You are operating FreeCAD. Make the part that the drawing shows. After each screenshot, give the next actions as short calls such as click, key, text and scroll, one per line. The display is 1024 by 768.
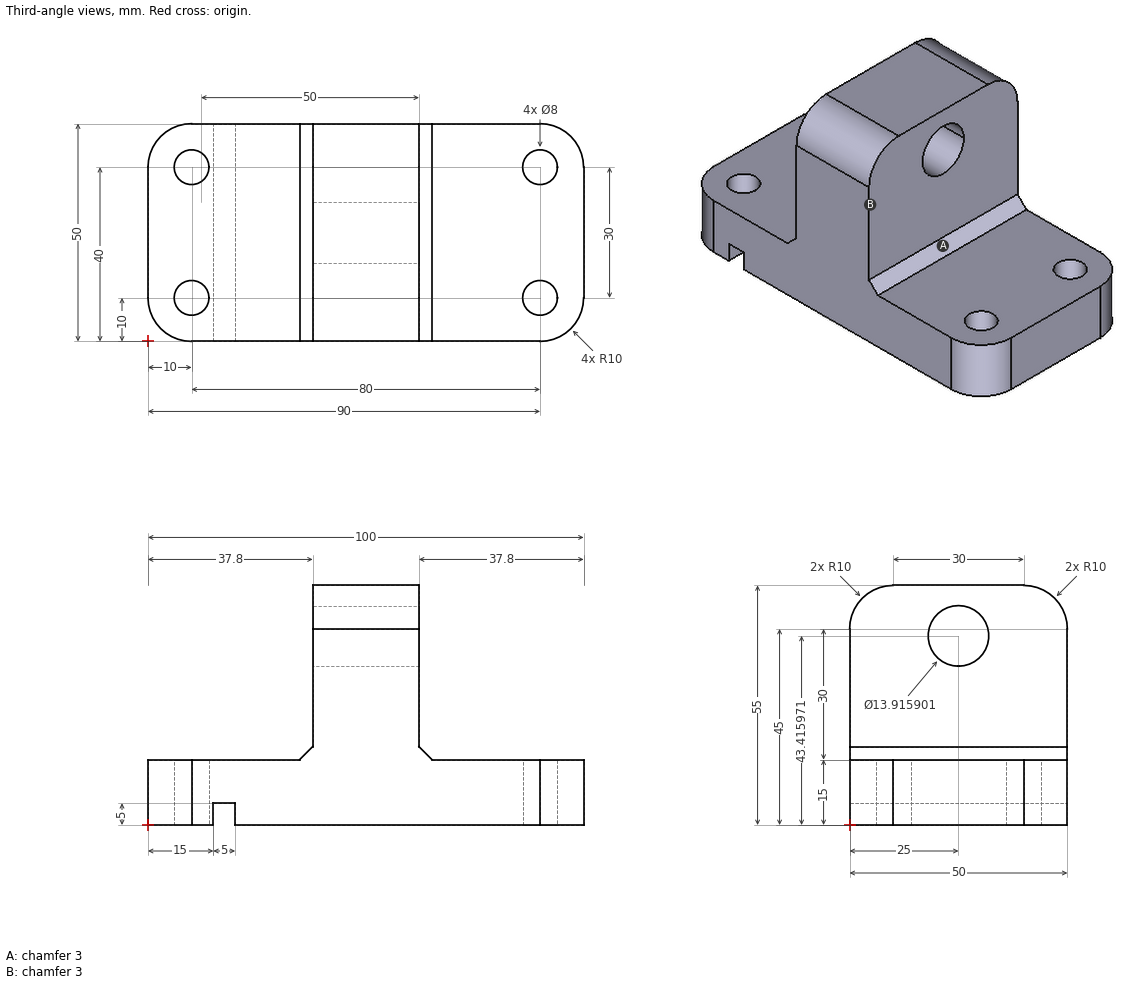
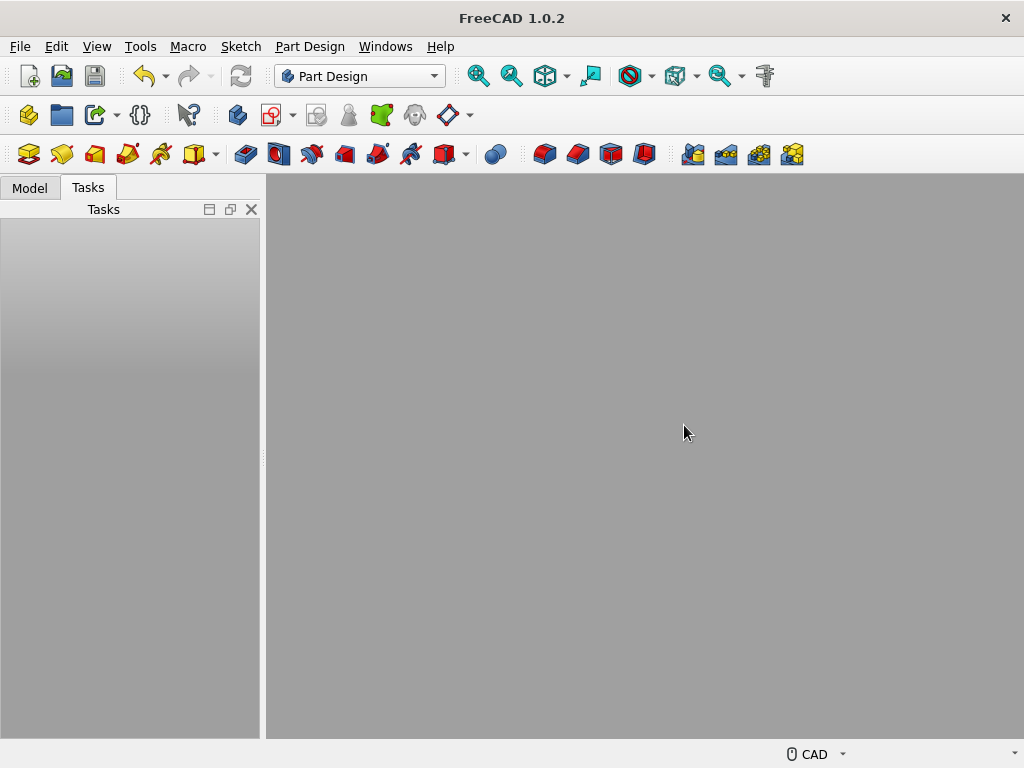
click(29, 76)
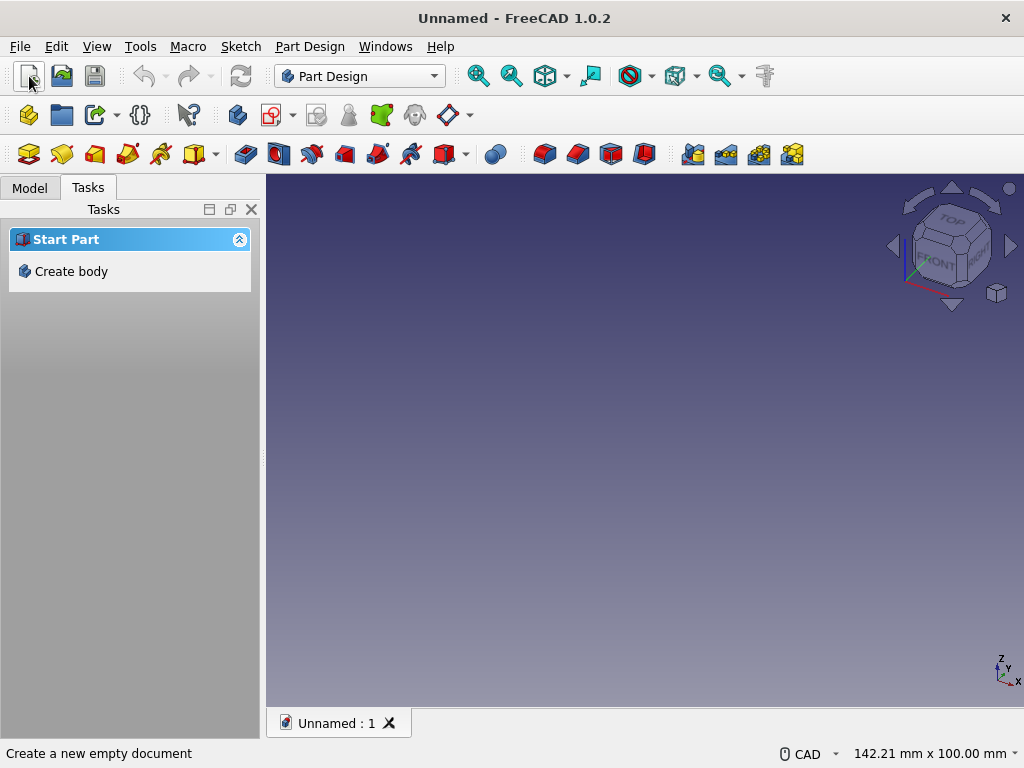
click(270, 116)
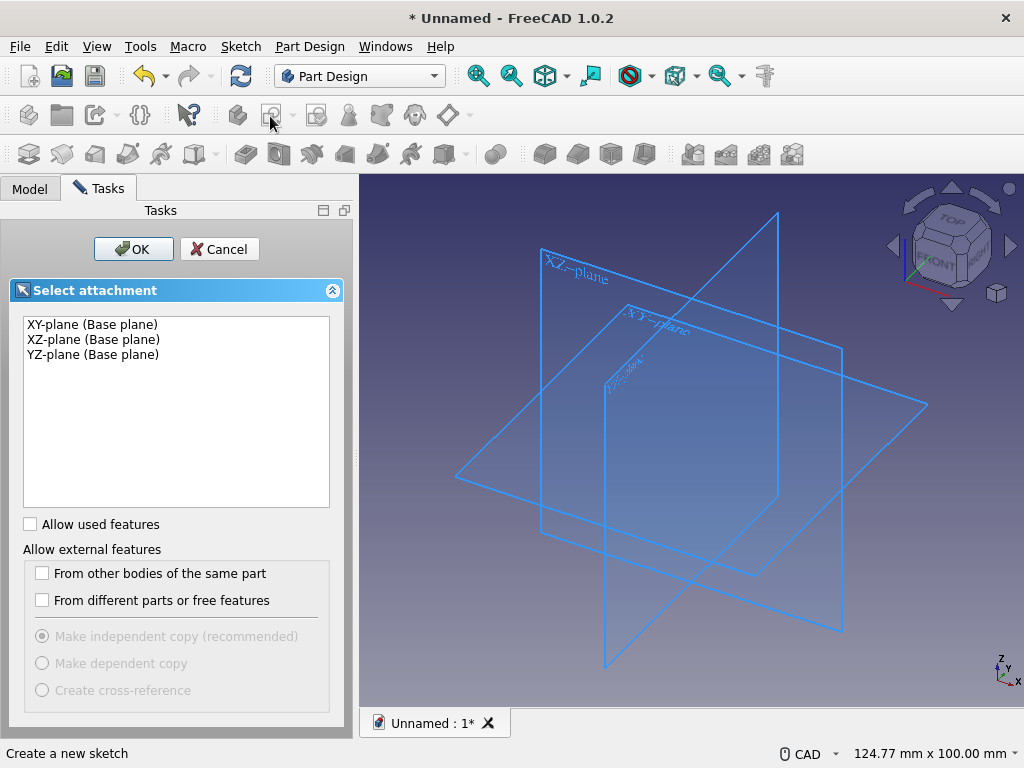
click(84, 324)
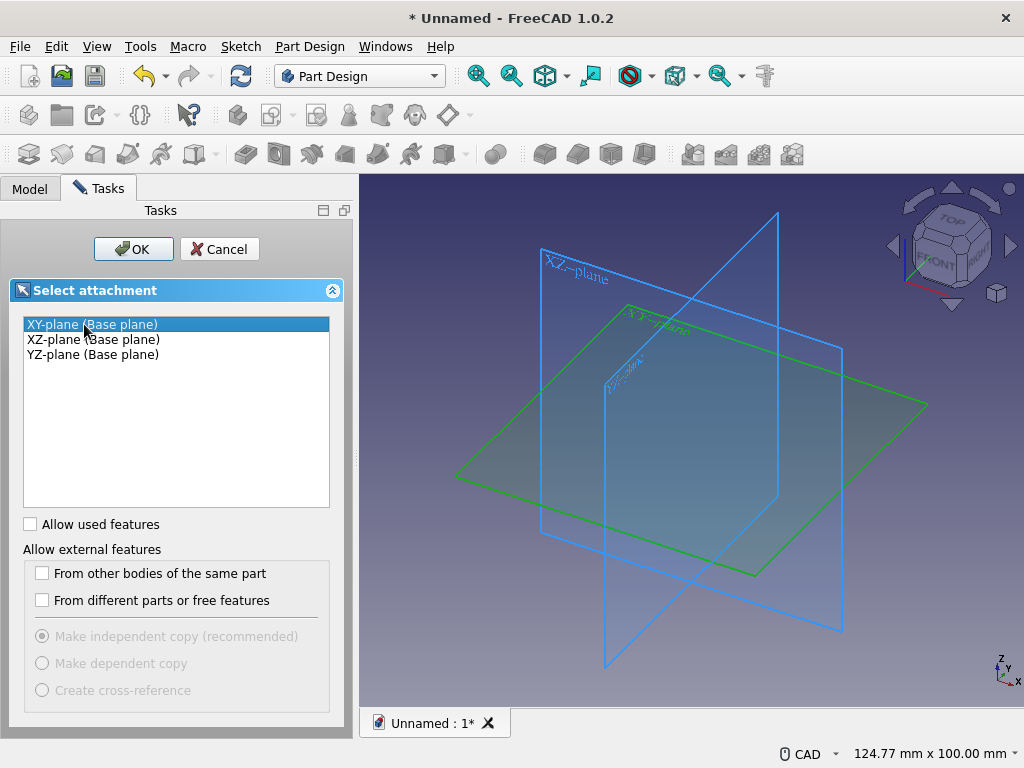
click(134, 249)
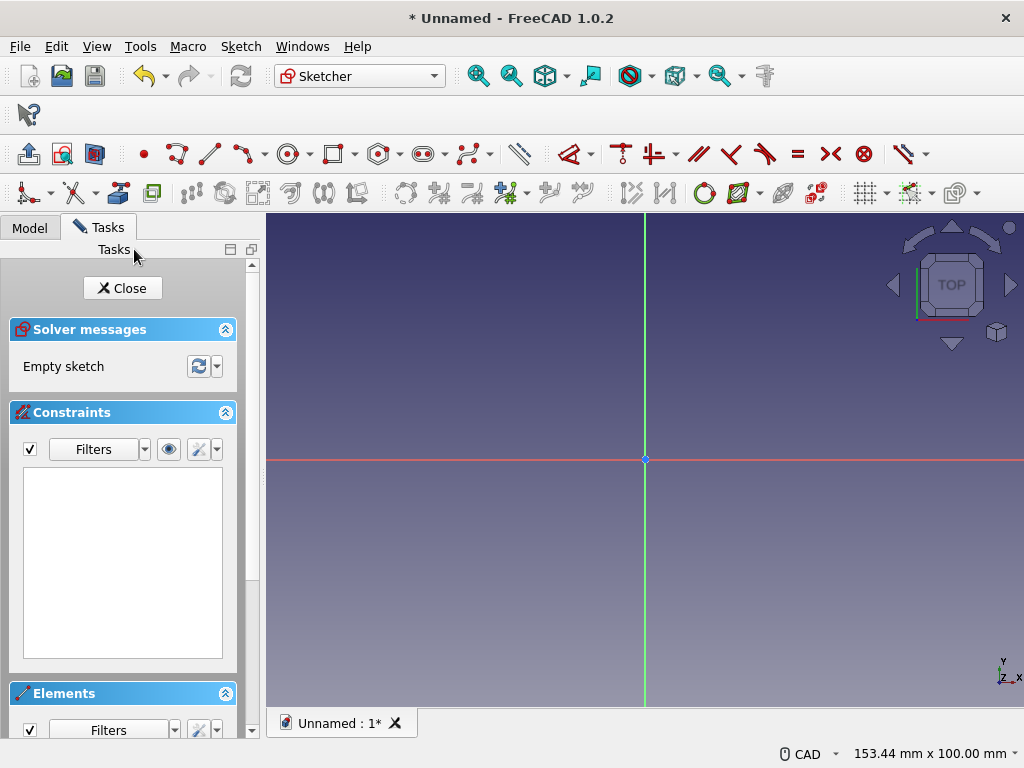
scroll(294, 610, down, 3)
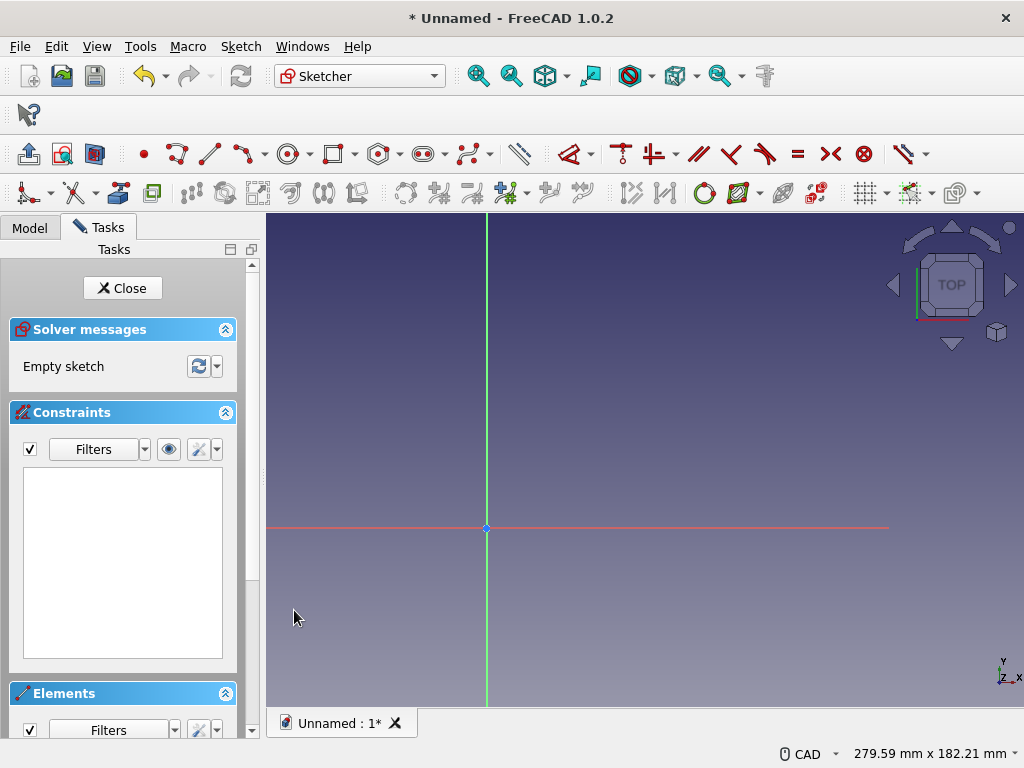
scroll(715, 461, up, 2)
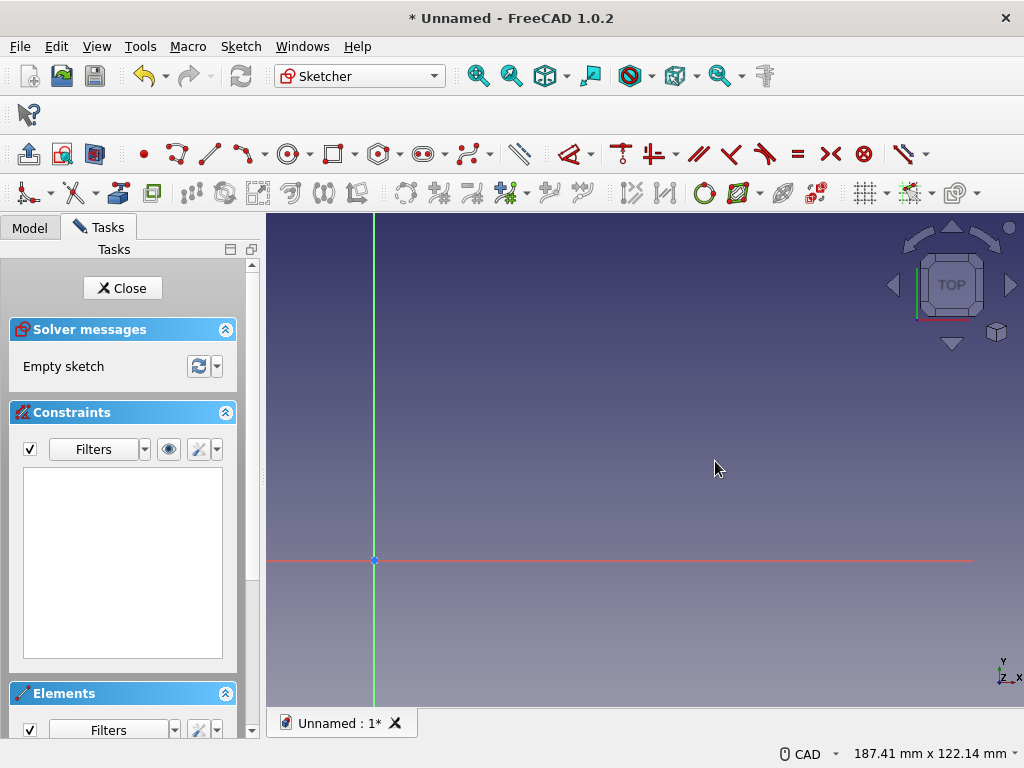
click(210, 154)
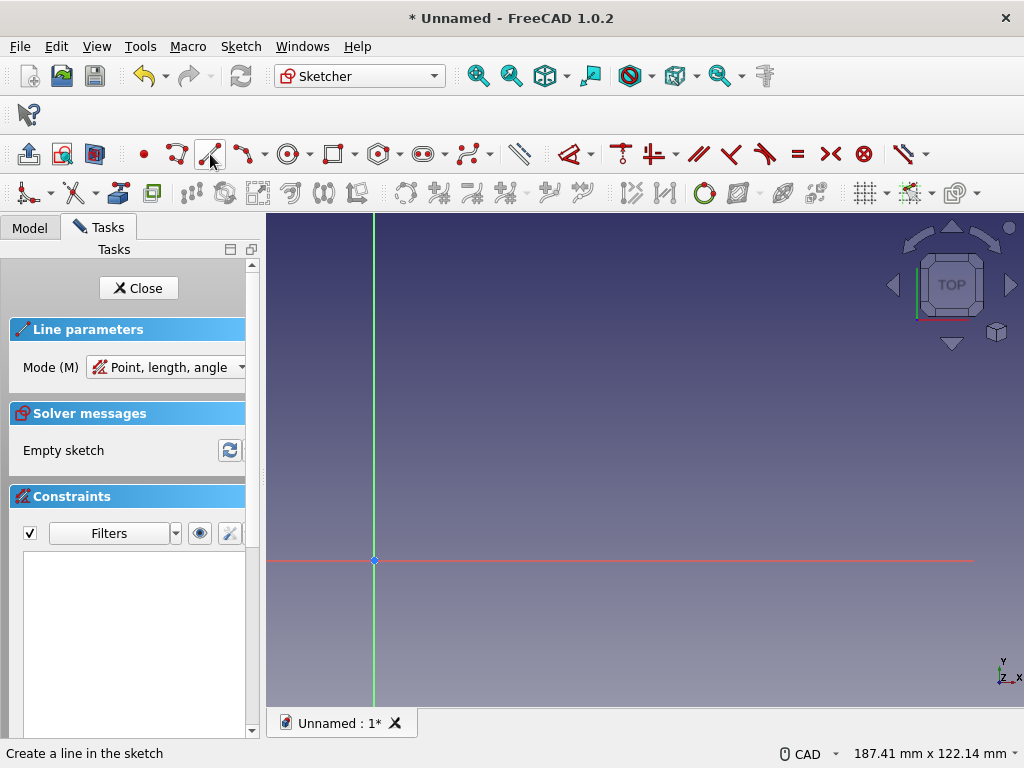
click(414, 561)
click(738, 552)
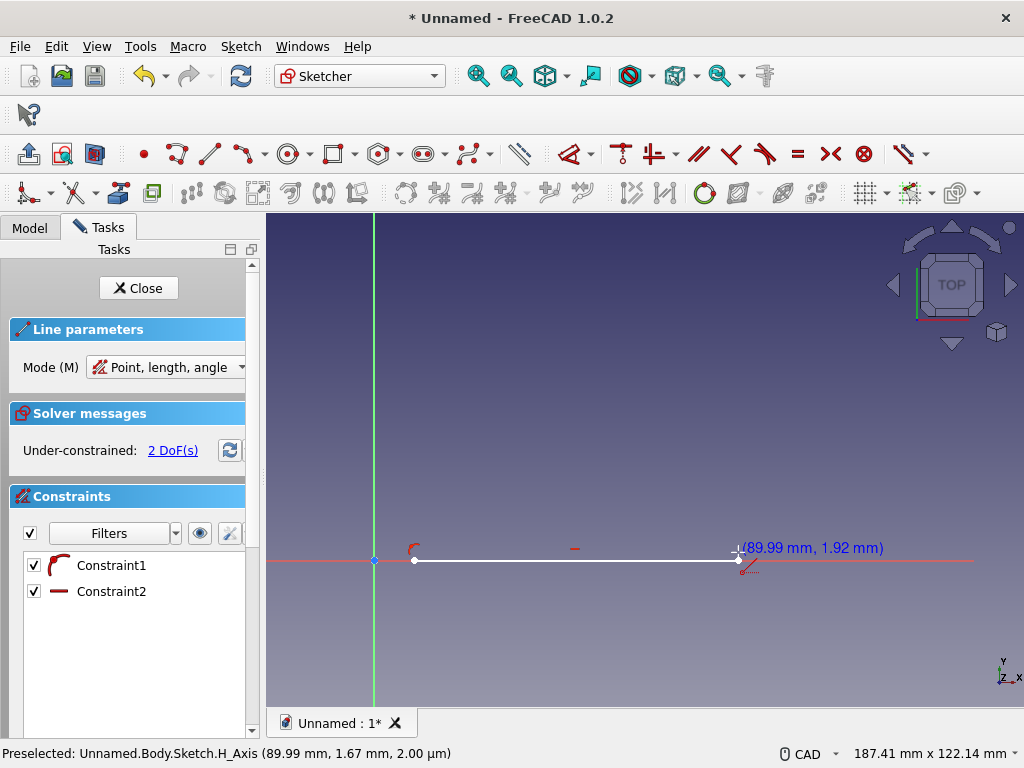
click(779, 520)
click(779, 399)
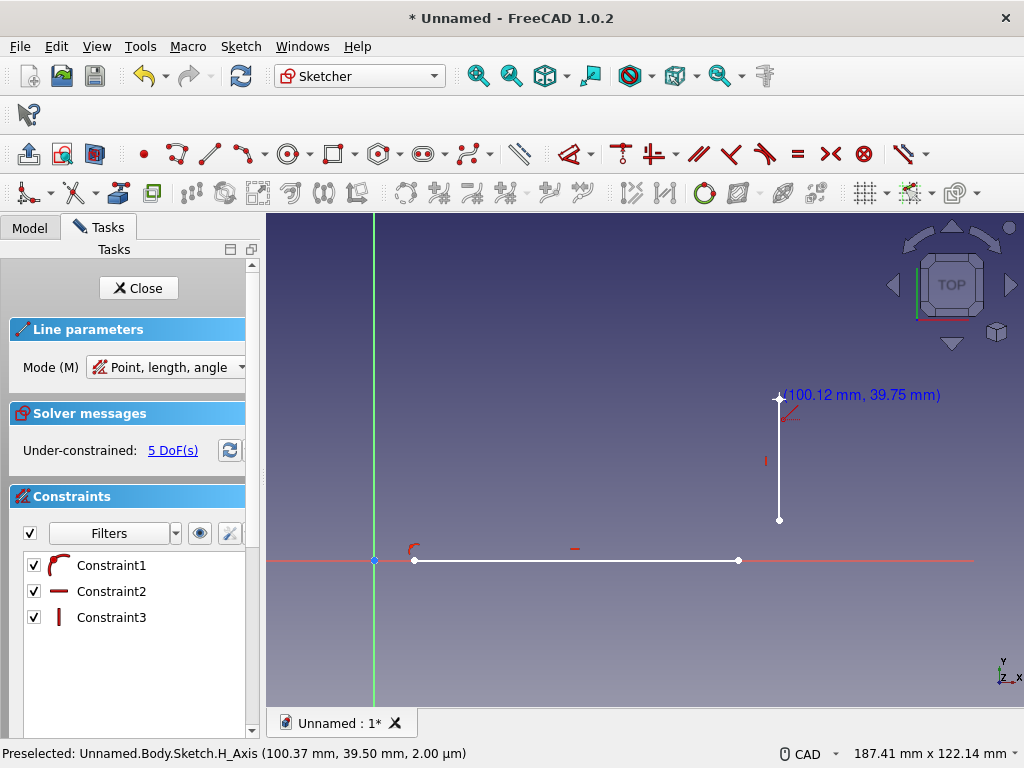
click(738, 359)
click(414, 359)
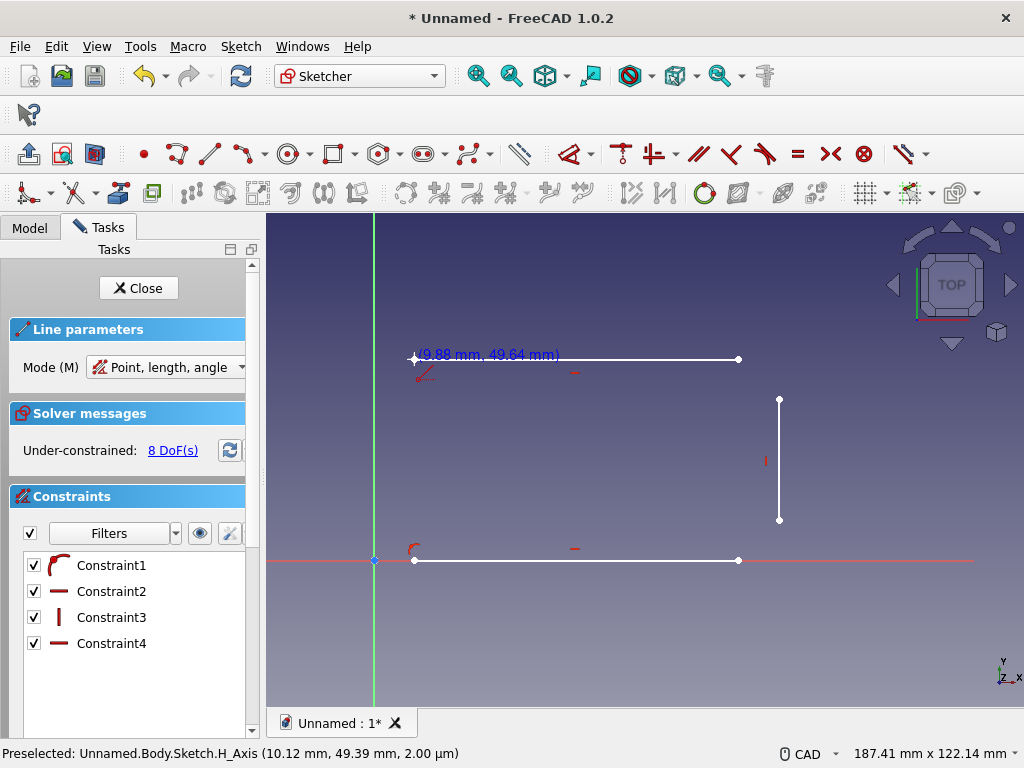
click(374, 399)
click(383, 520)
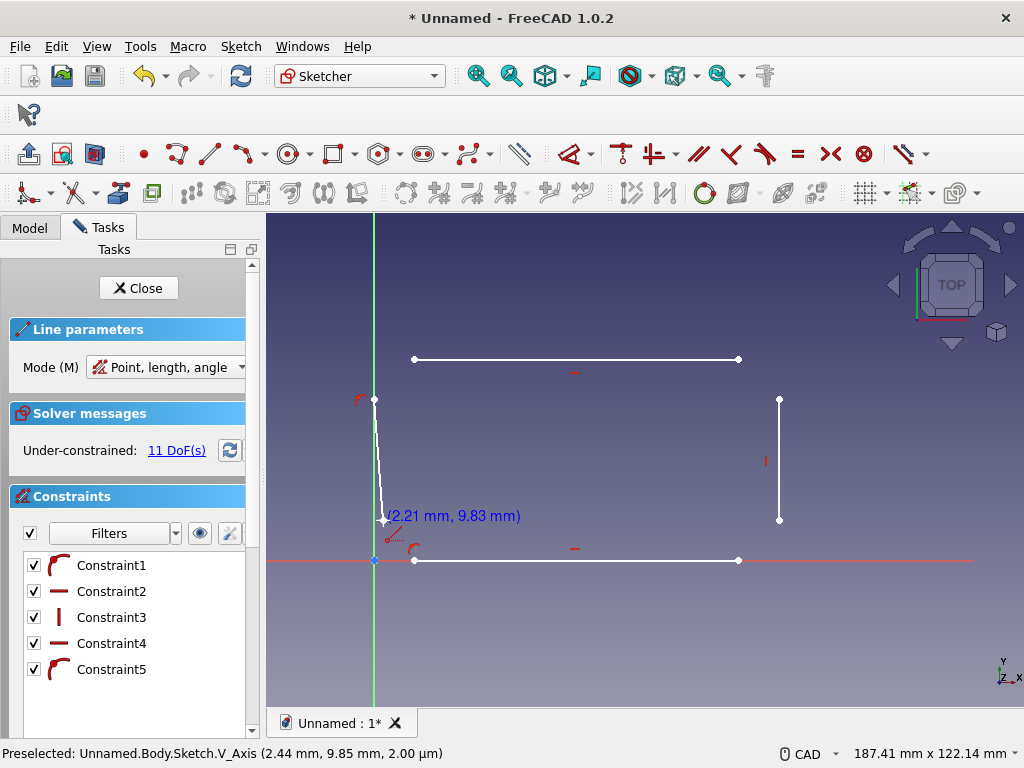
click(242, 154)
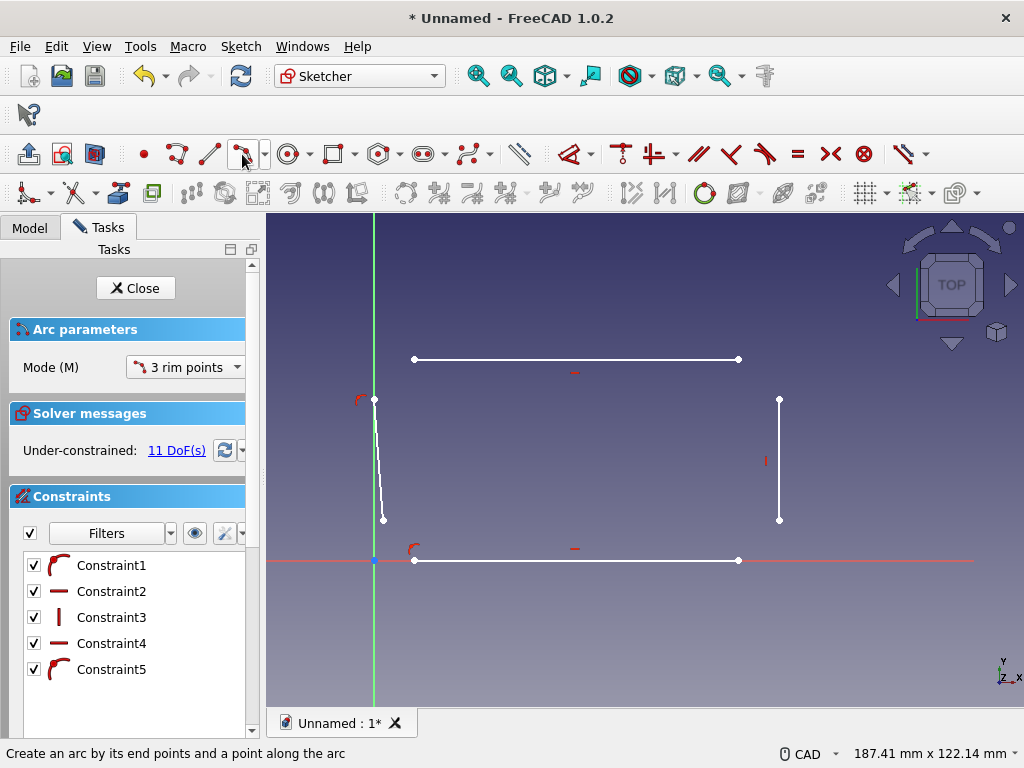
click(738, 561)
click(779, 521)